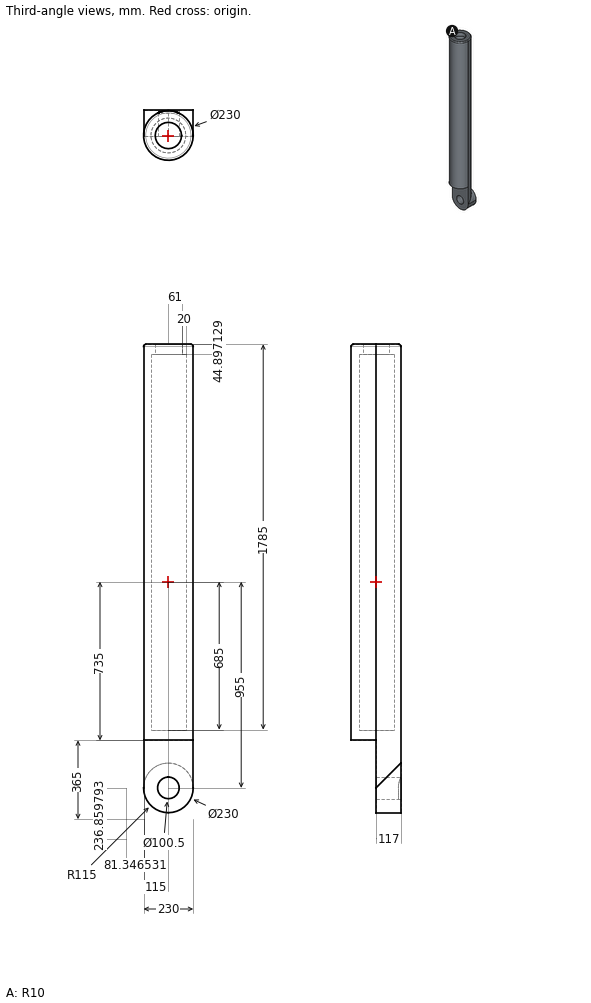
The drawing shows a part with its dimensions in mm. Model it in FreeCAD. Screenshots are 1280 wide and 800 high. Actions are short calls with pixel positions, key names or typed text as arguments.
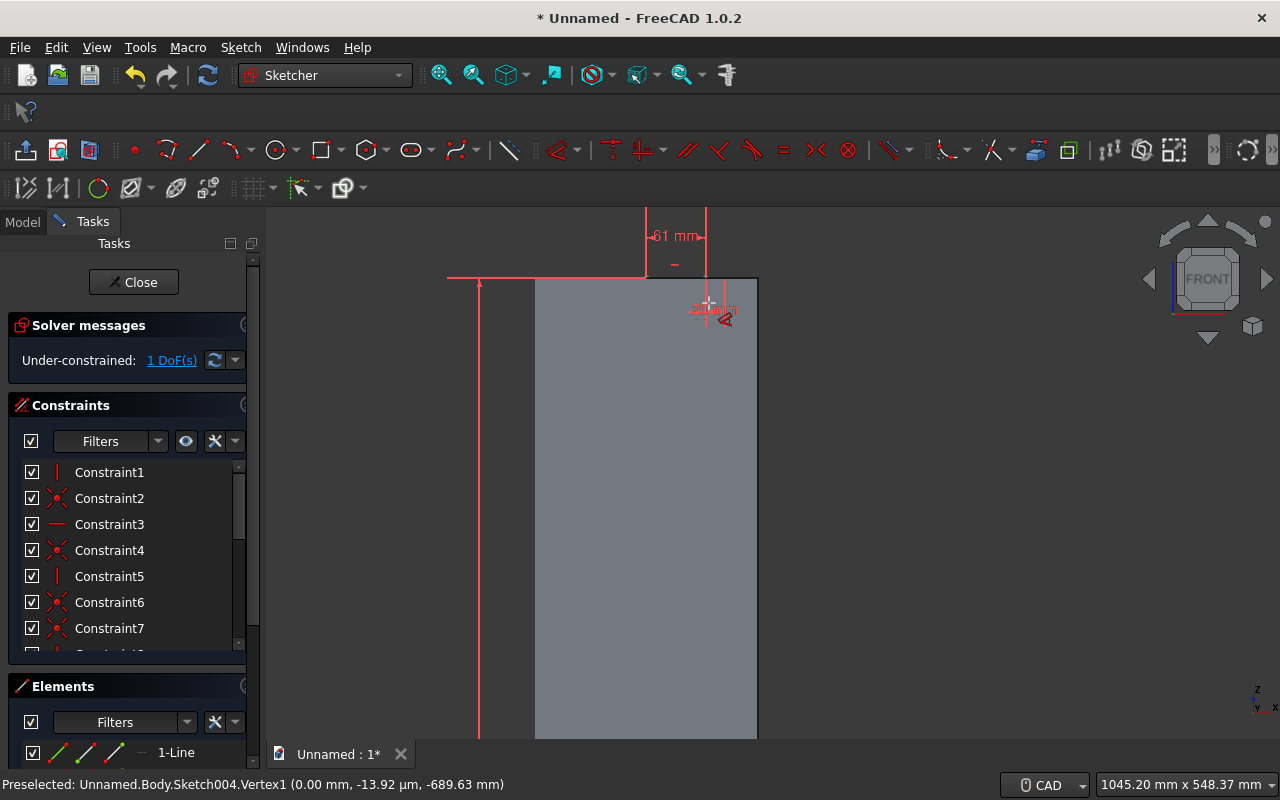
click(706, 302)
click(740, 291)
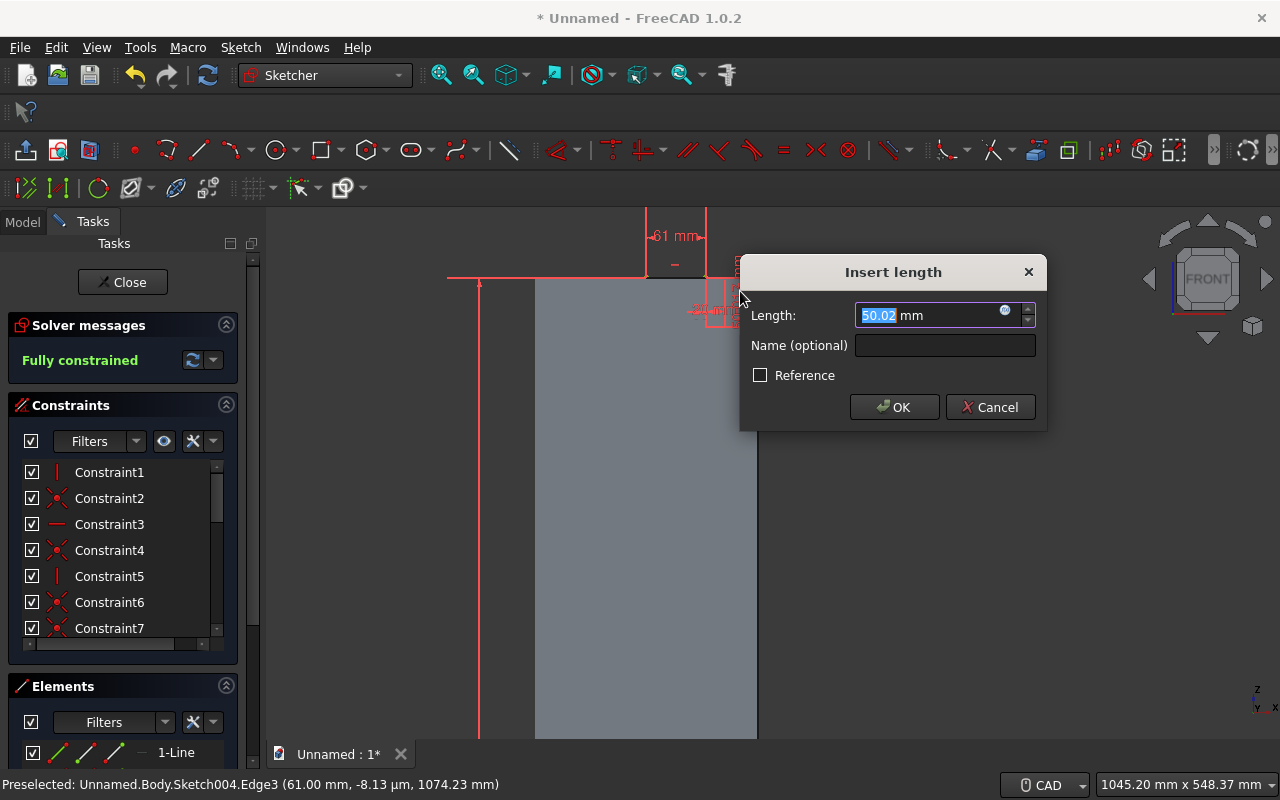
text(44.897129)
key(Return)
key(Escape)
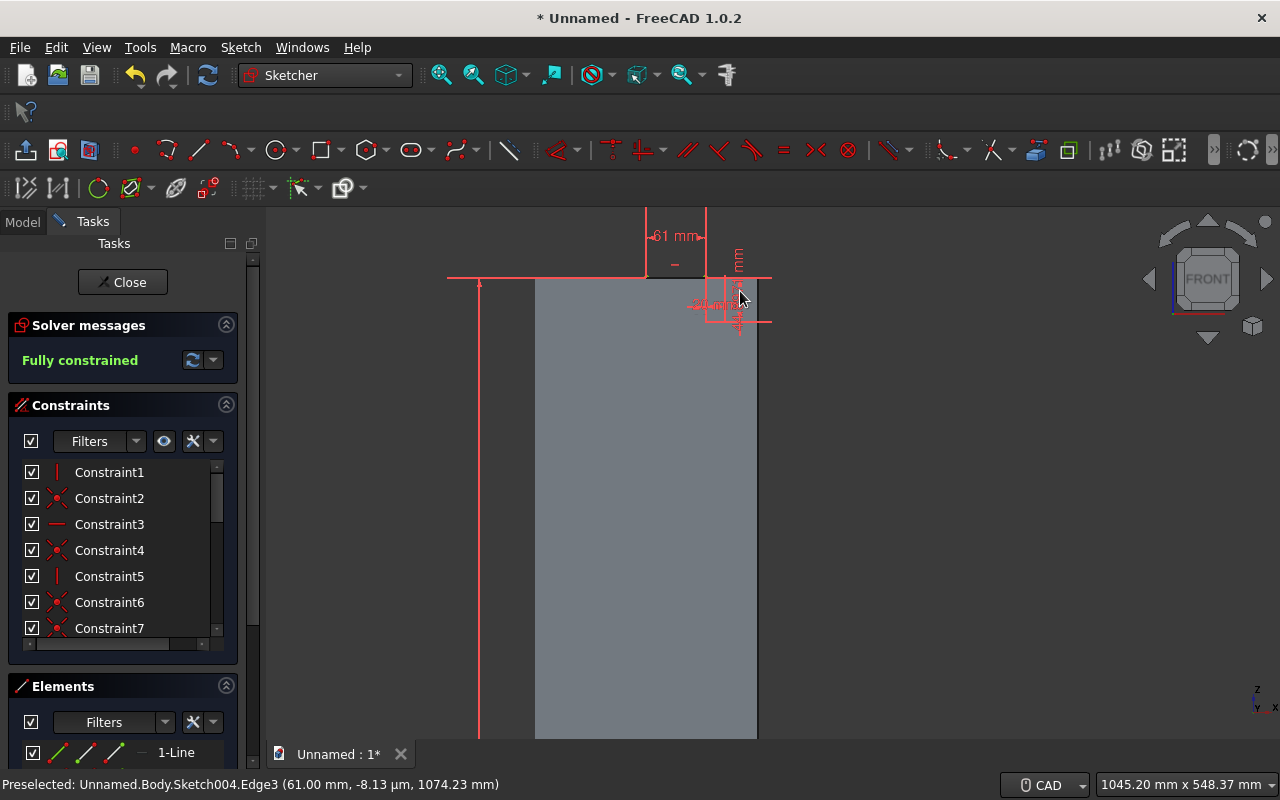
click(123, 282)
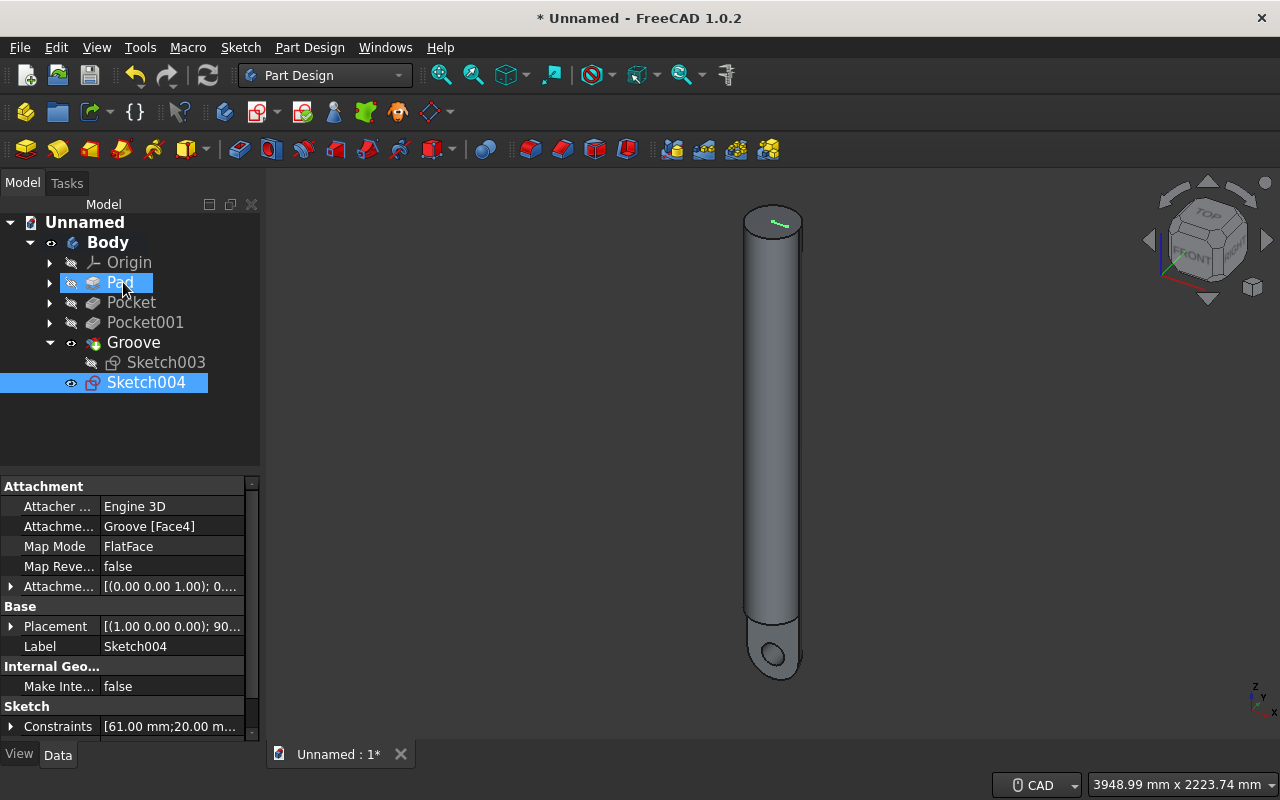
click(304, 150)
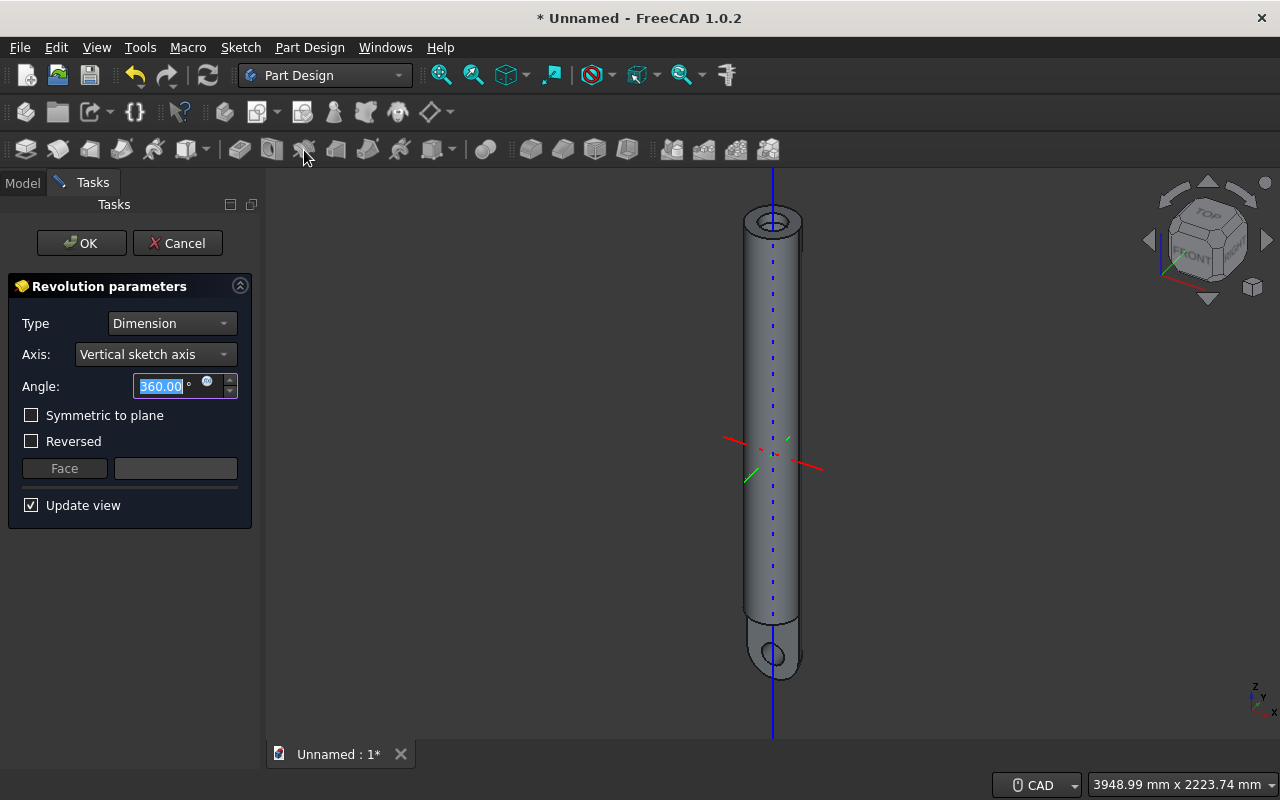
click(82, 243)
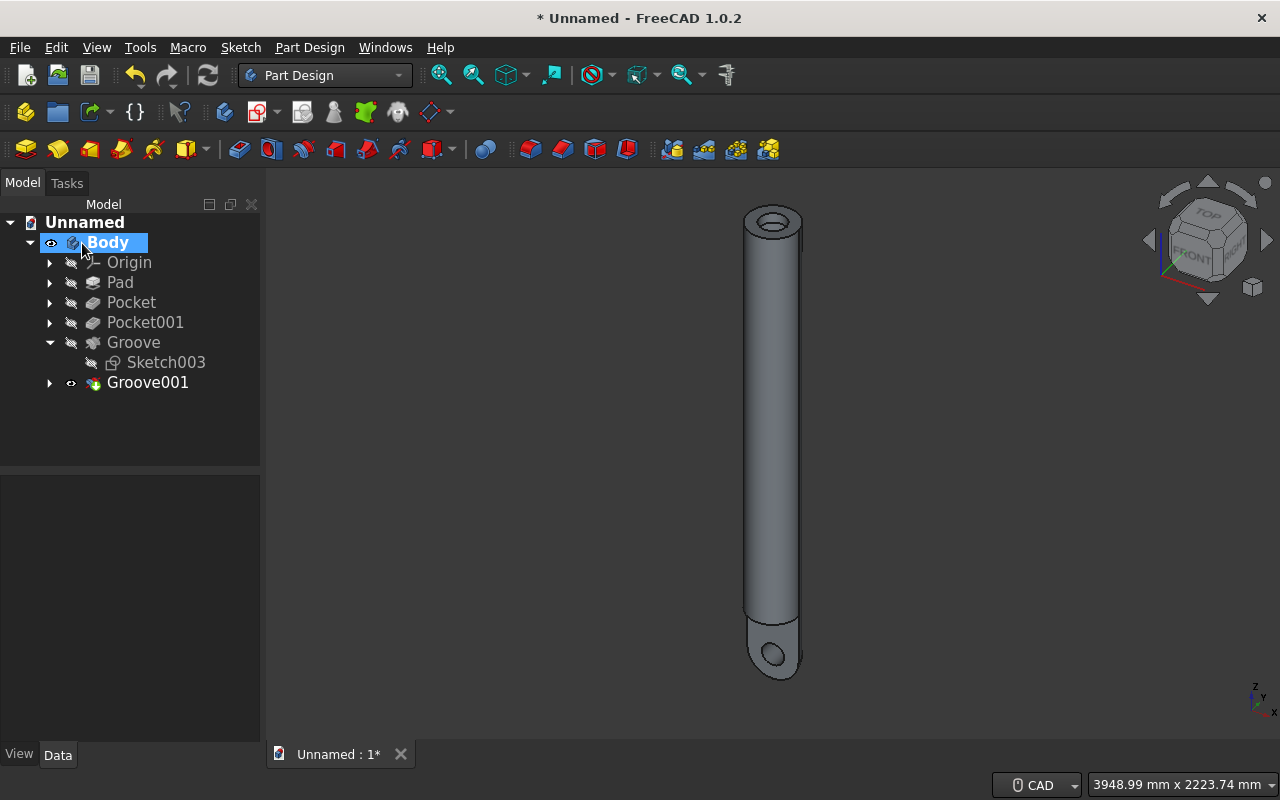
click(50, 263)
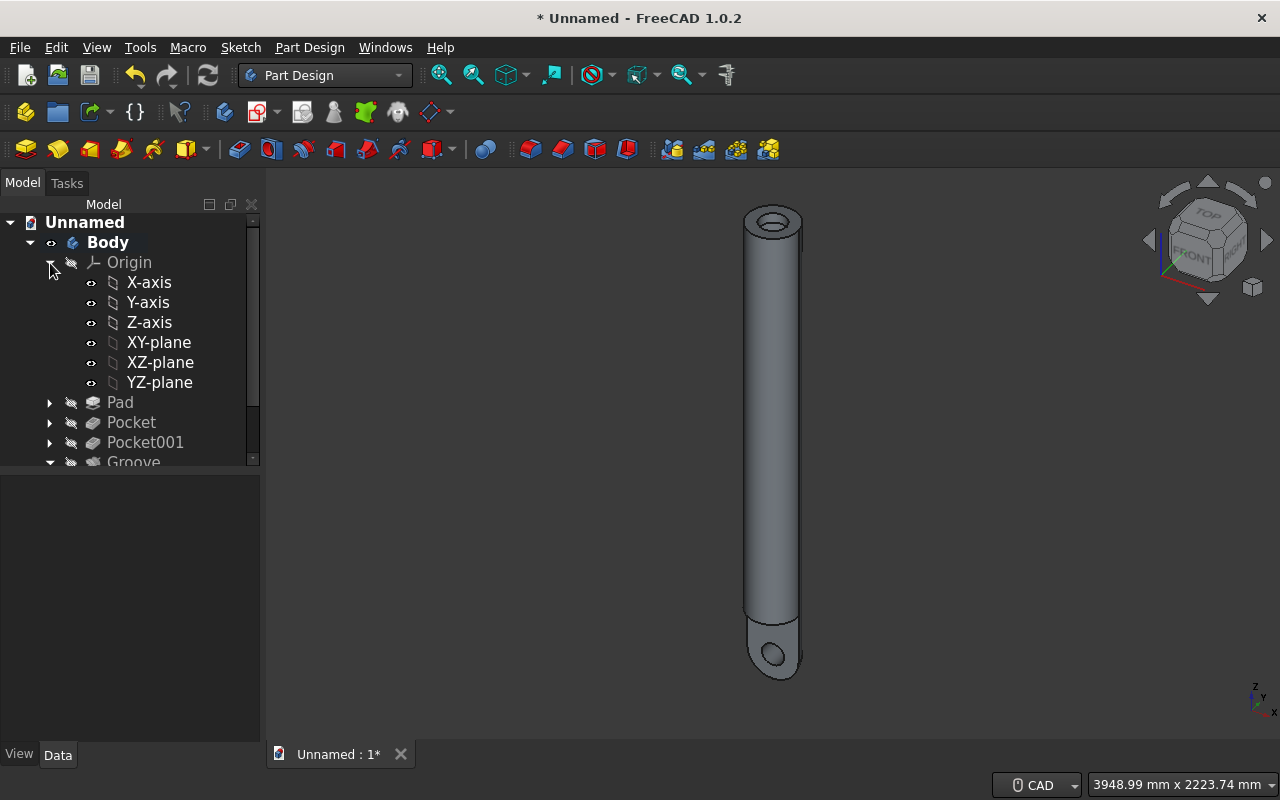
click(136, 363)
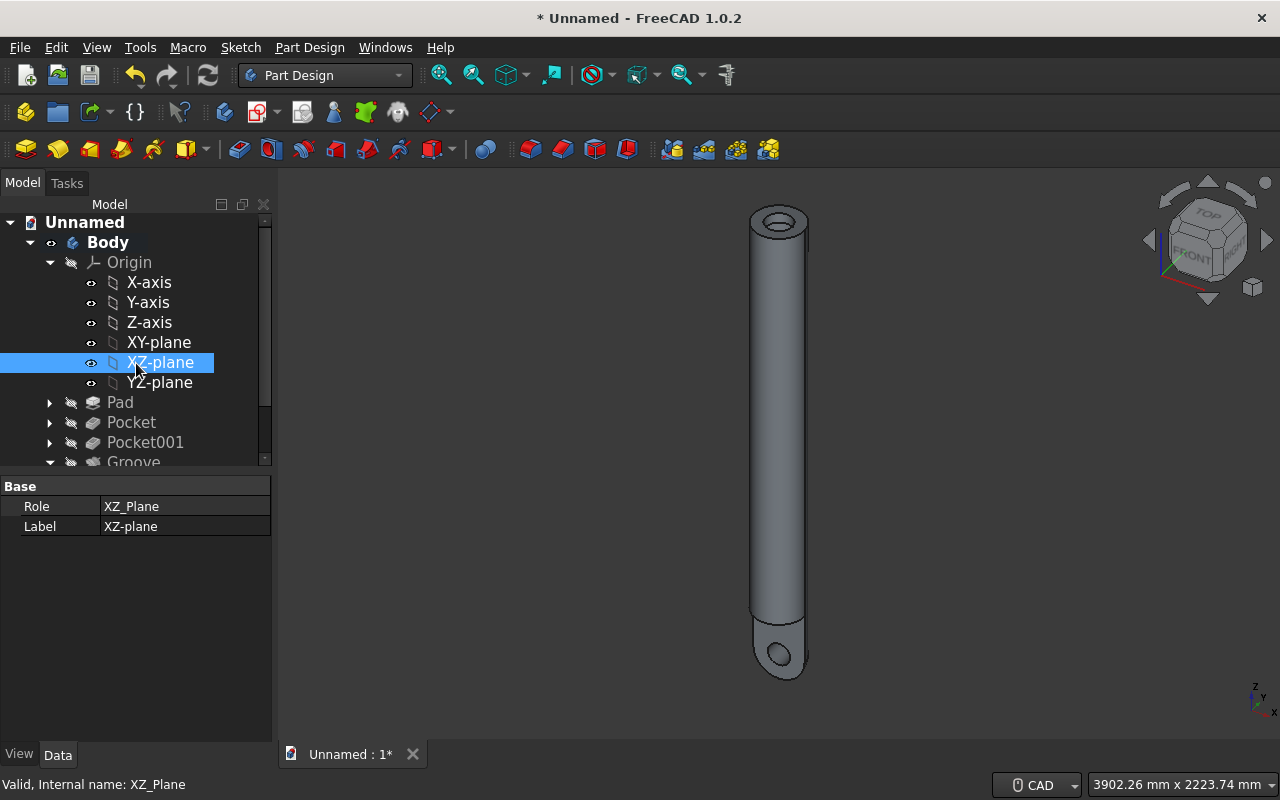
click(430, 112)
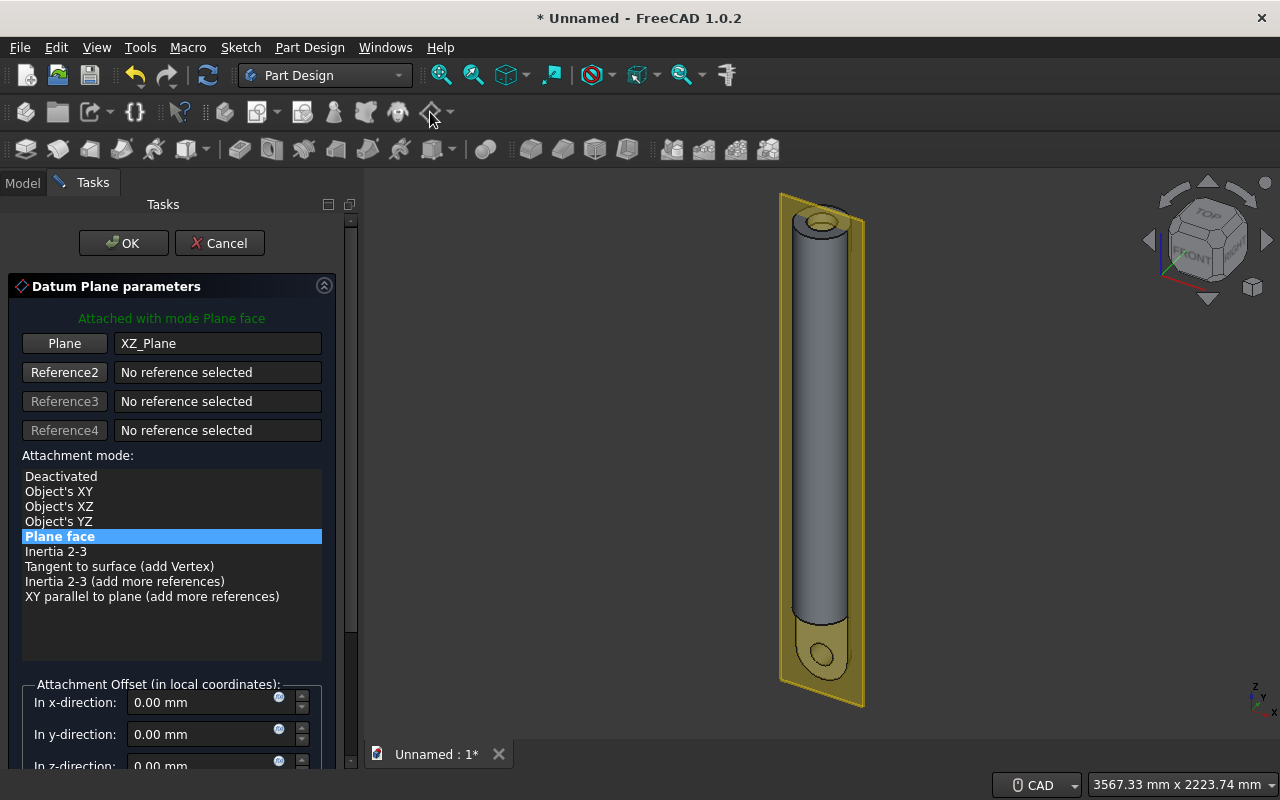
scroll(351, 491, down, 2)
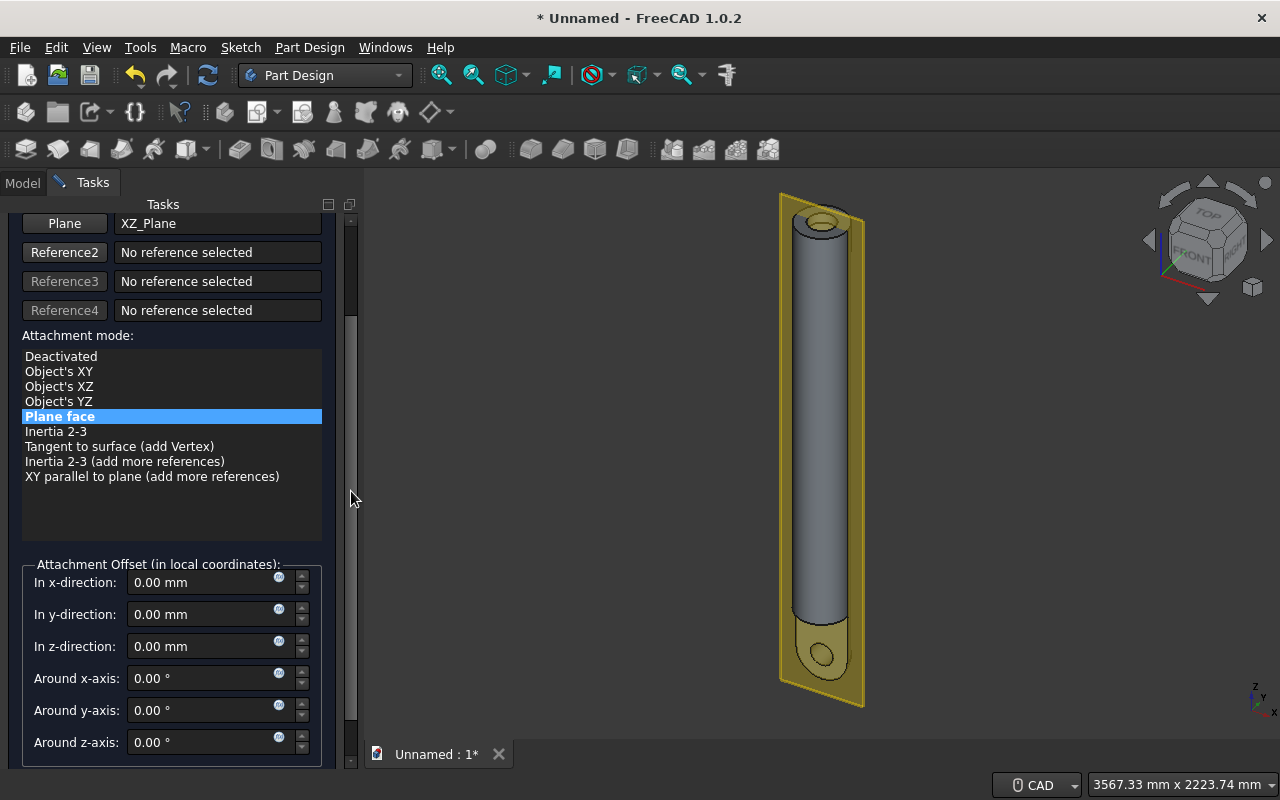
triple_click(210, 646)